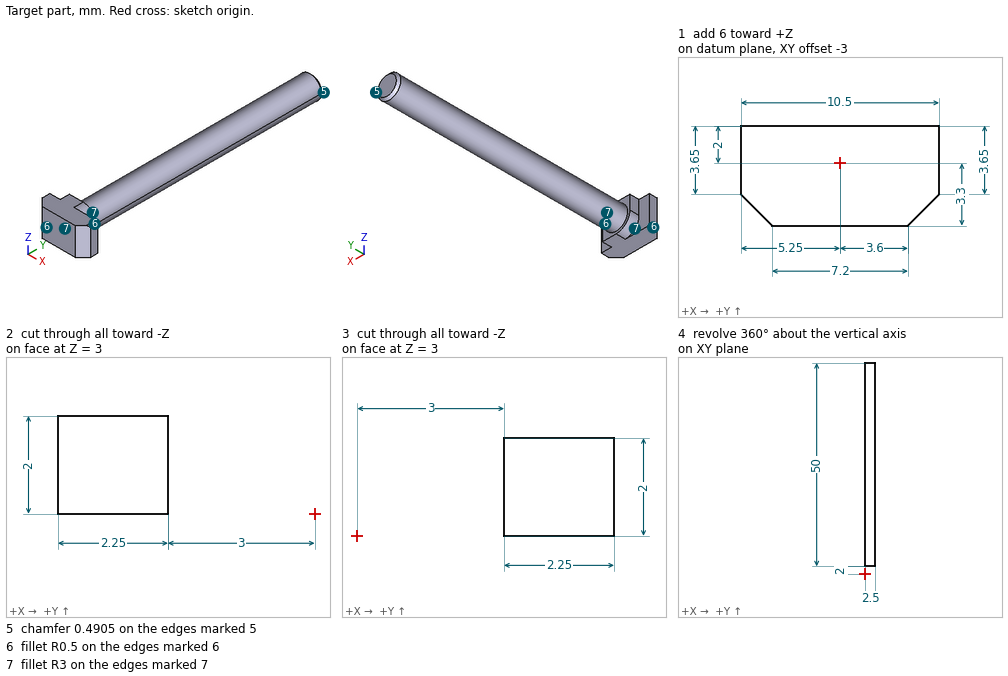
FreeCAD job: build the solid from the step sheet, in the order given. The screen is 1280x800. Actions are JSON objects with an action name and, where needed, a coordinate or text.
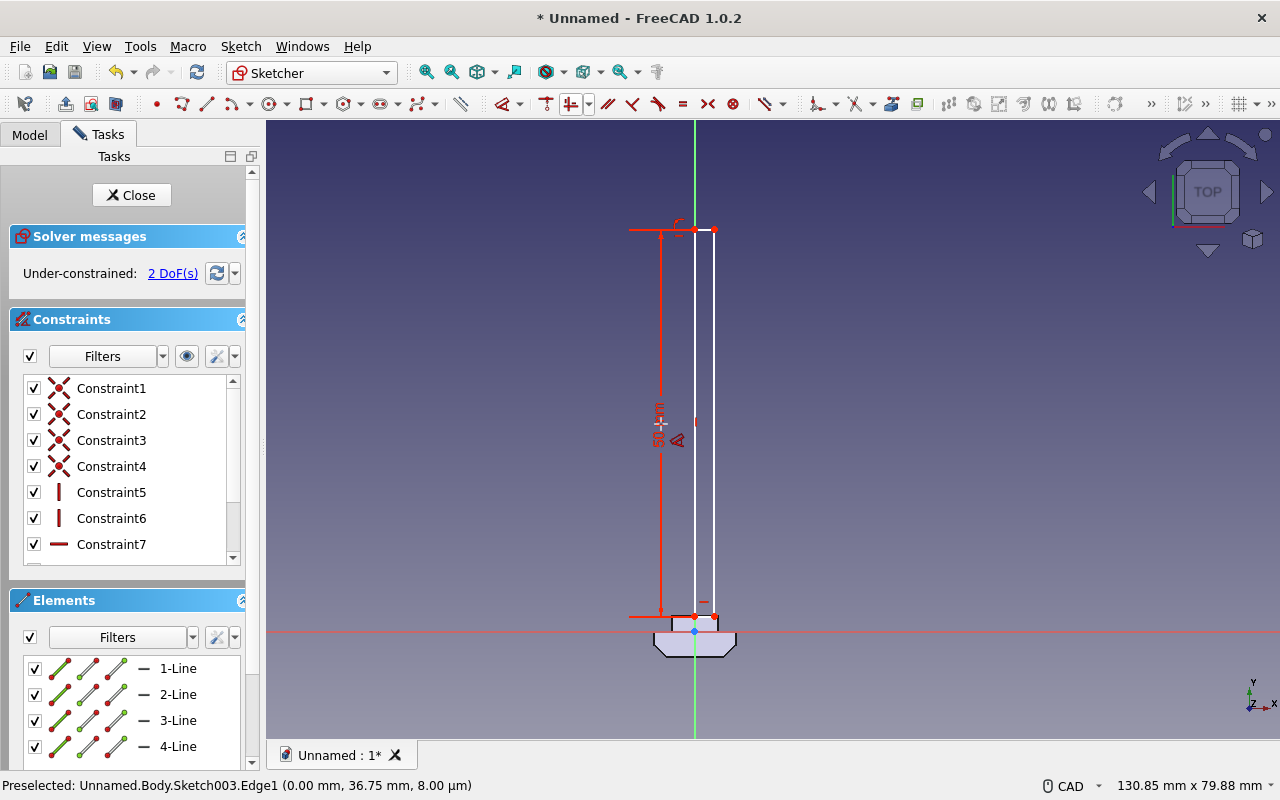
{"action": "scroll", "coordinate": [695, 617], "scroll_direction": "up", "scroll_amount": 5}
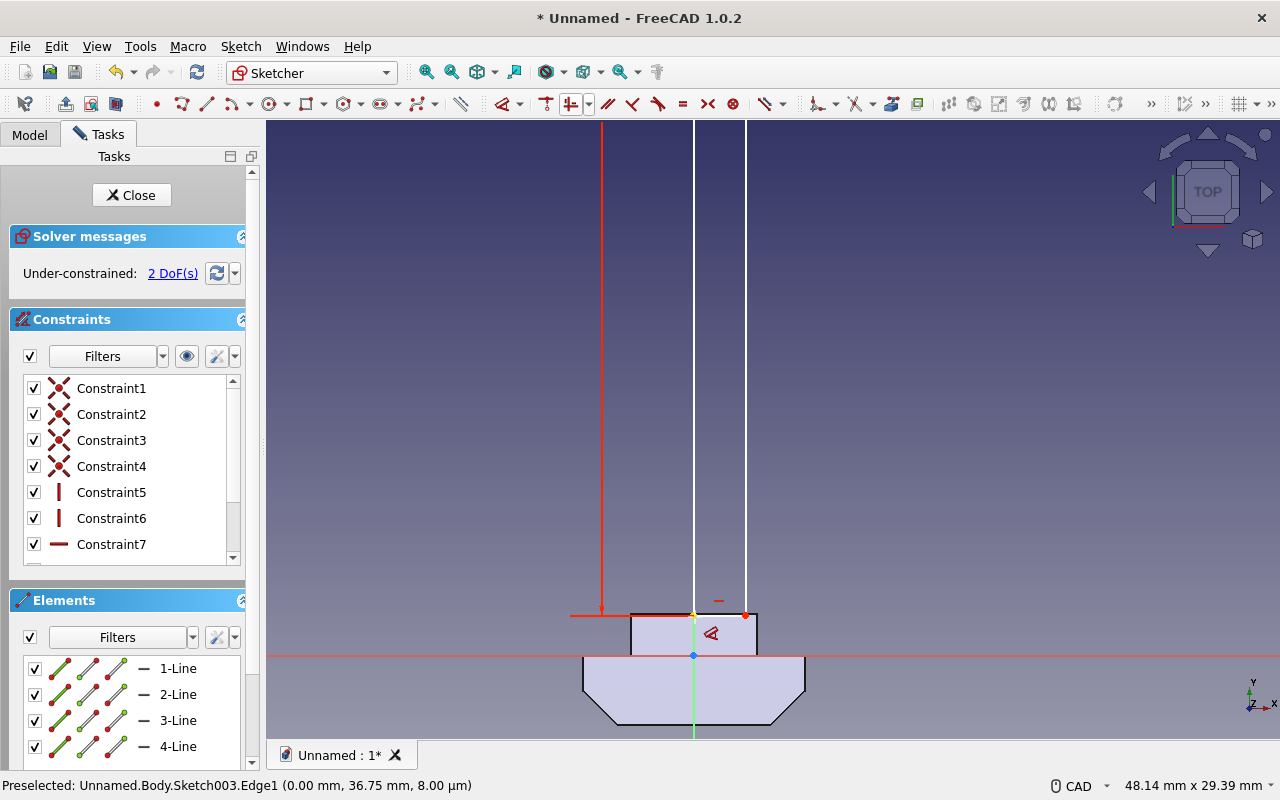
{"action": "left_click", "coordinate": [694, 616]}
{"action": "left_click", "coordinate": [660, 636]}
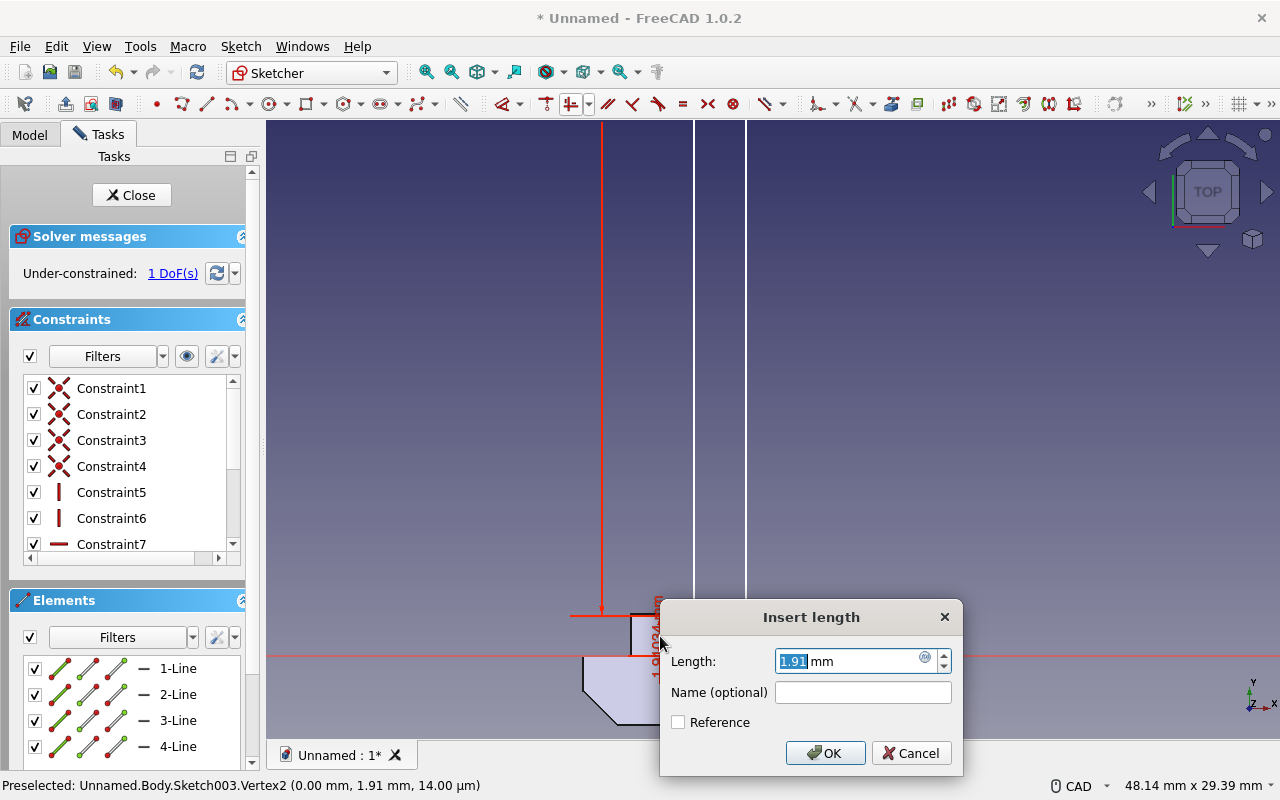
{"action": "type", "text": "2"}
{"action": "key", "text": "Return"}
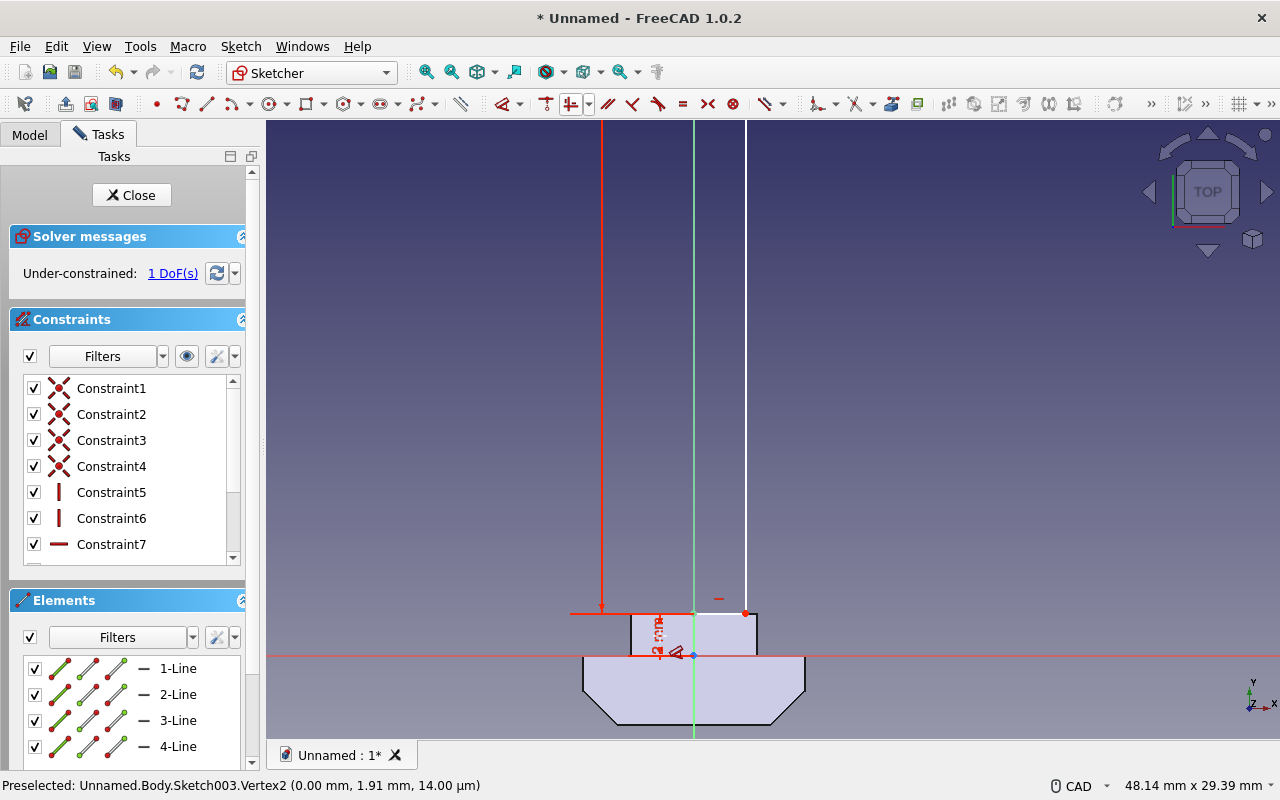
{"action": "left_click", "coordinate": [710, 614]}
{"action": "left_click", "coordinate": [720, 580]}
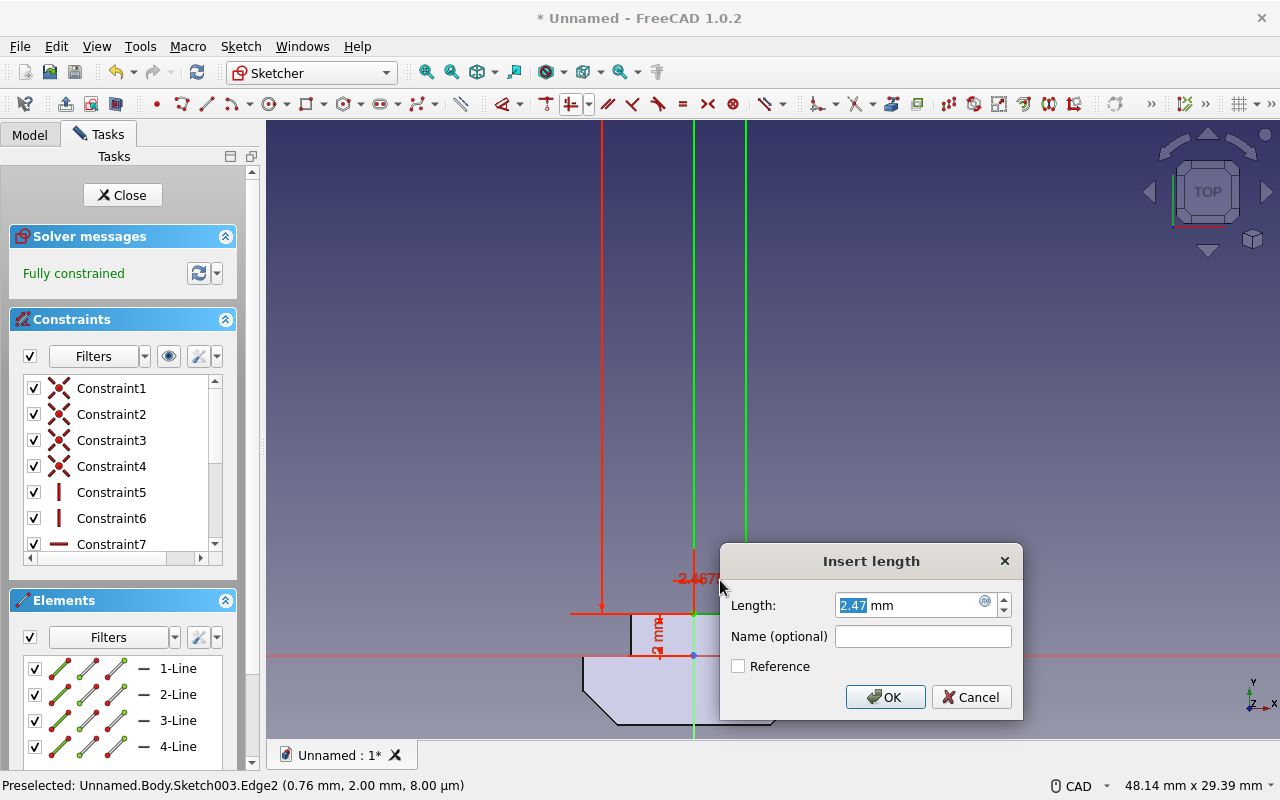
{"action": "type", "text": "2.5"}
{"action": "key", "text": "Return"}
{"action": "key", "text": "Escape"}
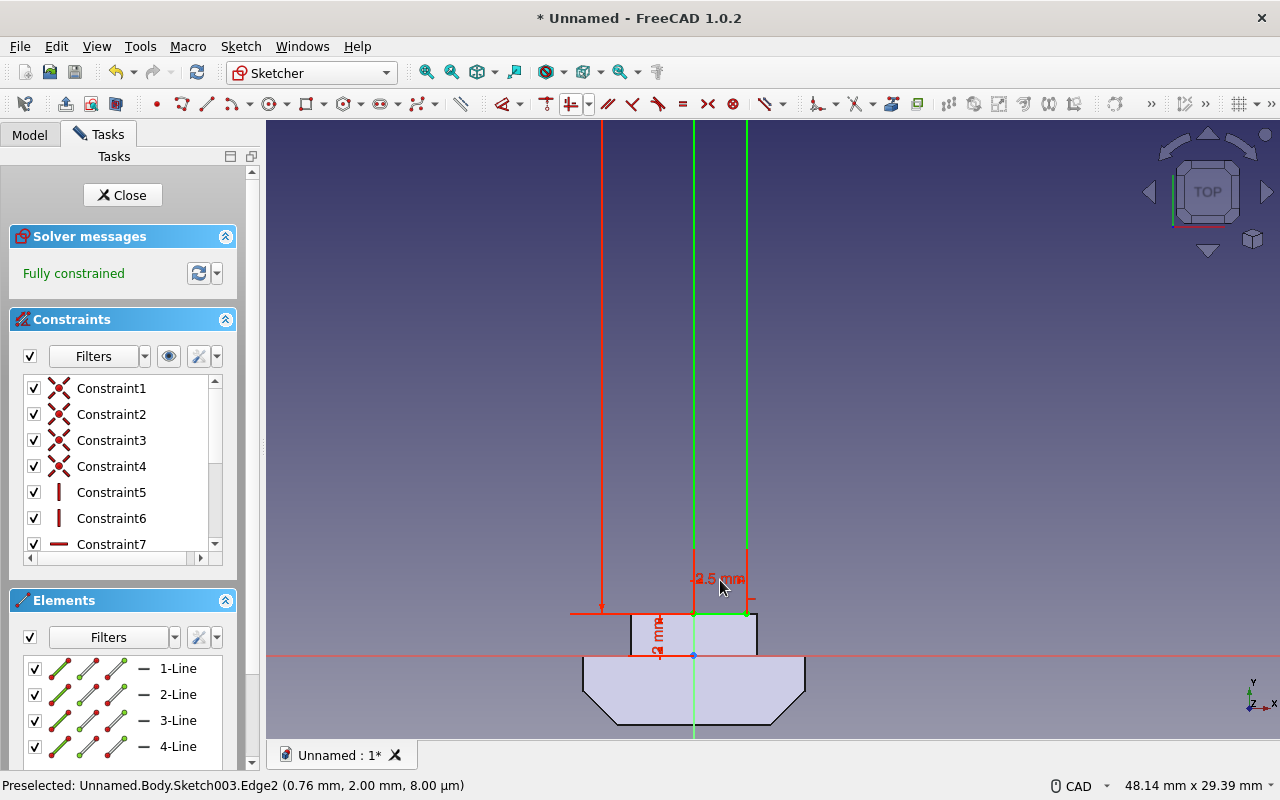
{"action": "left_click", "coordinate": [123, 195]}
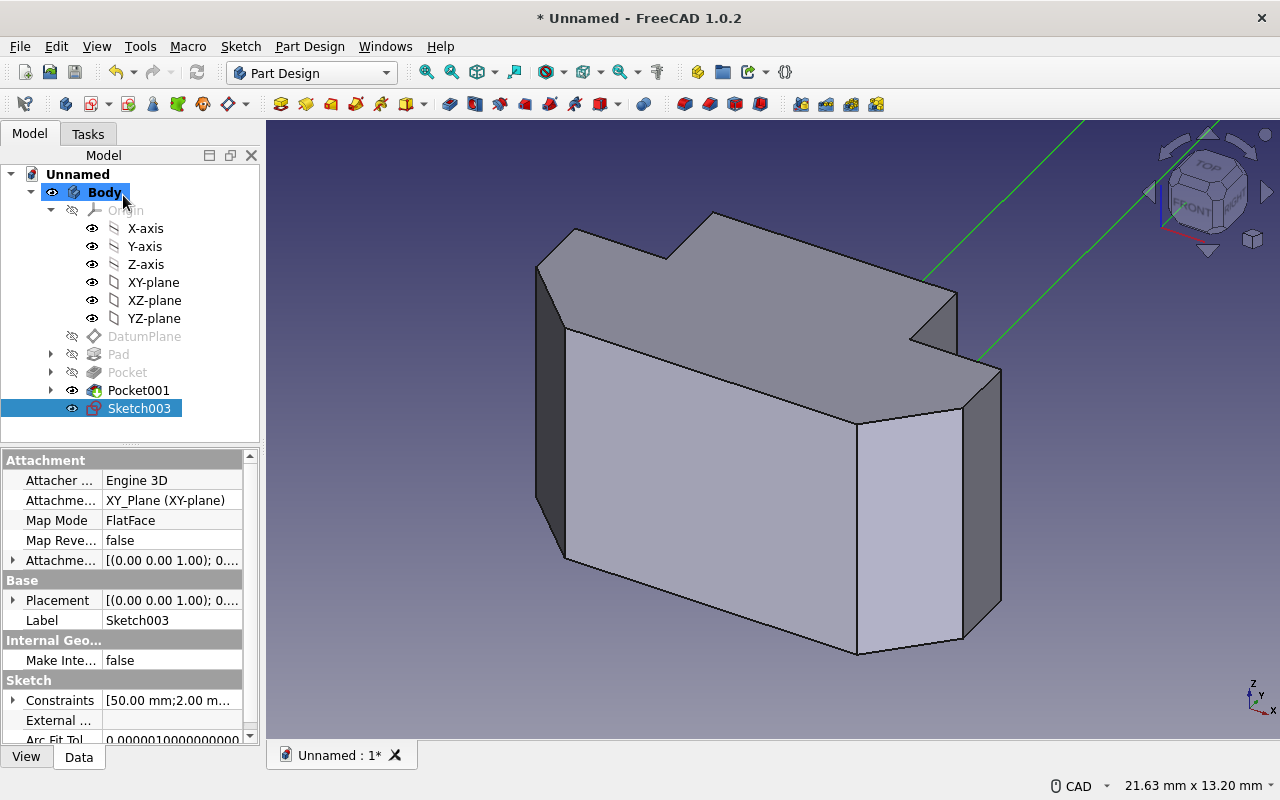
{"action": "left_click", "coordinate": [306, 104]}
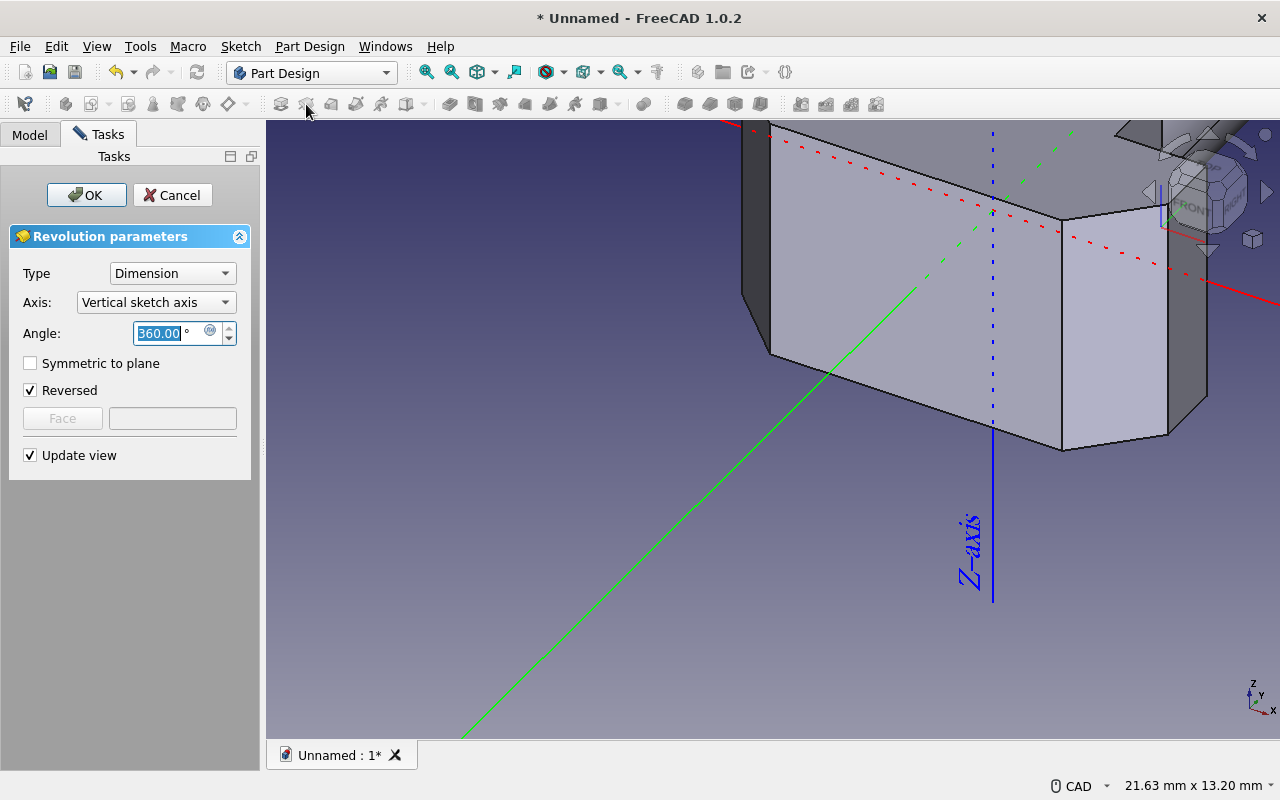
{"action": "left_click", "coordinate": [87, 195]}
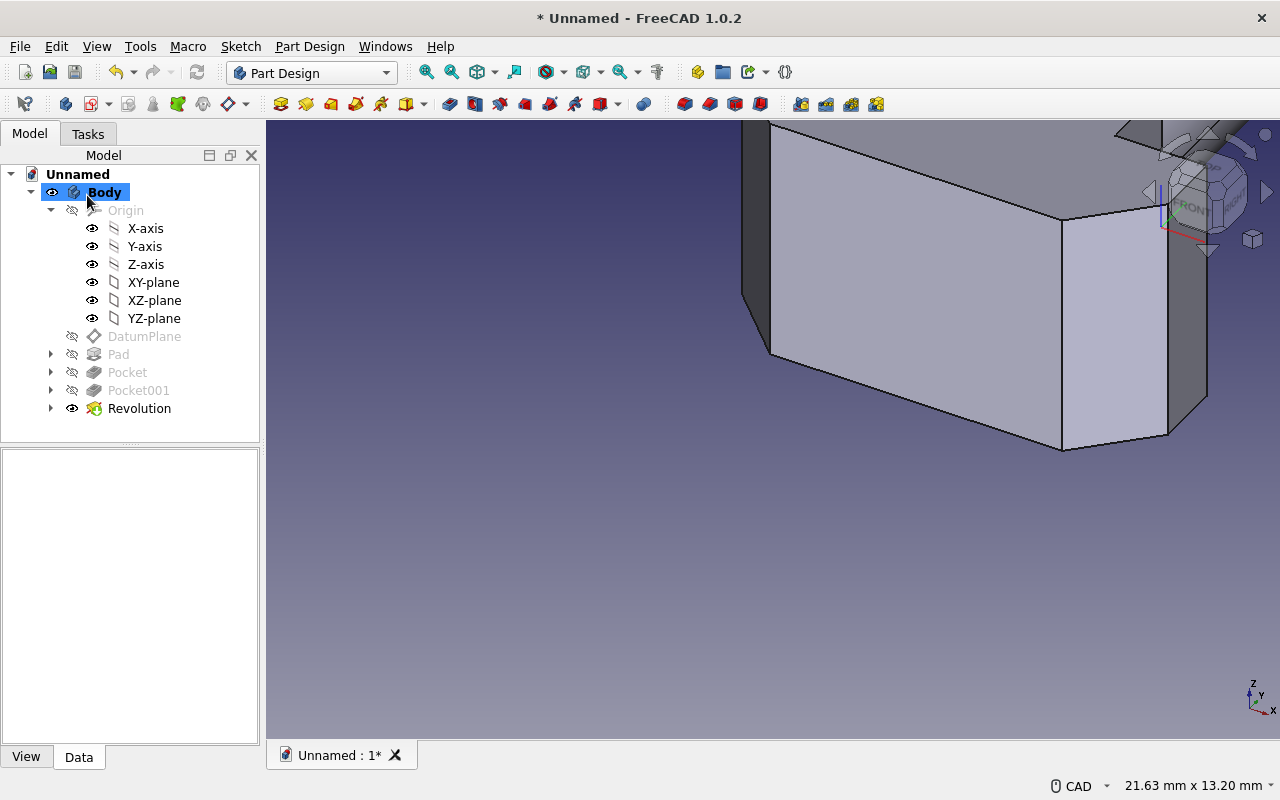
{"action": "key", "text": "v f"}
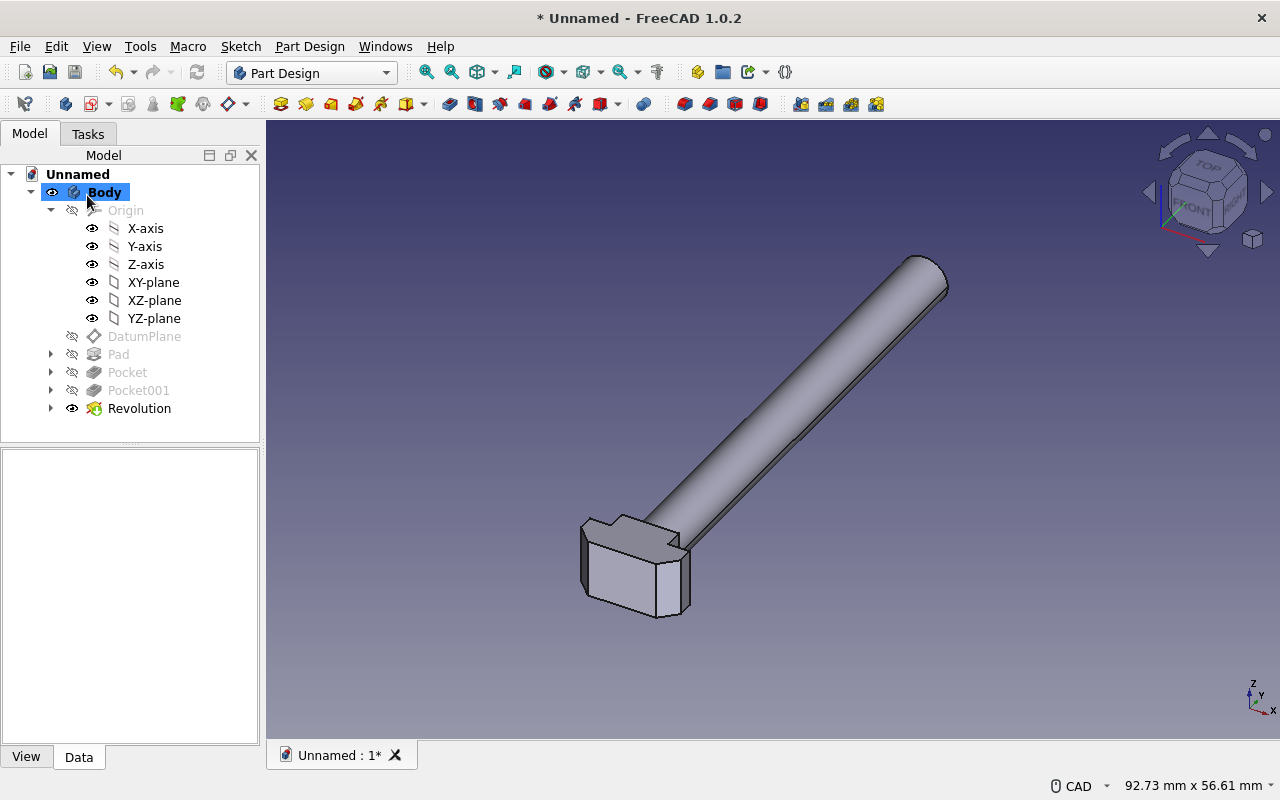
{"action": "key", "text": "0"}